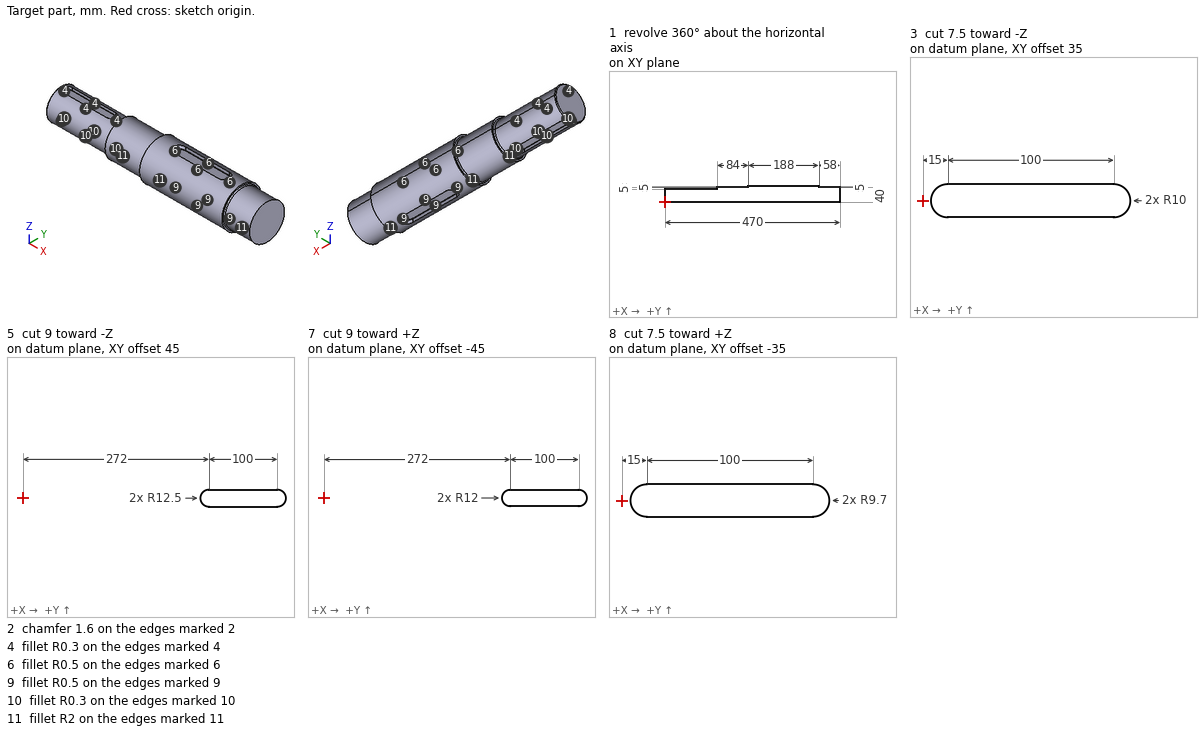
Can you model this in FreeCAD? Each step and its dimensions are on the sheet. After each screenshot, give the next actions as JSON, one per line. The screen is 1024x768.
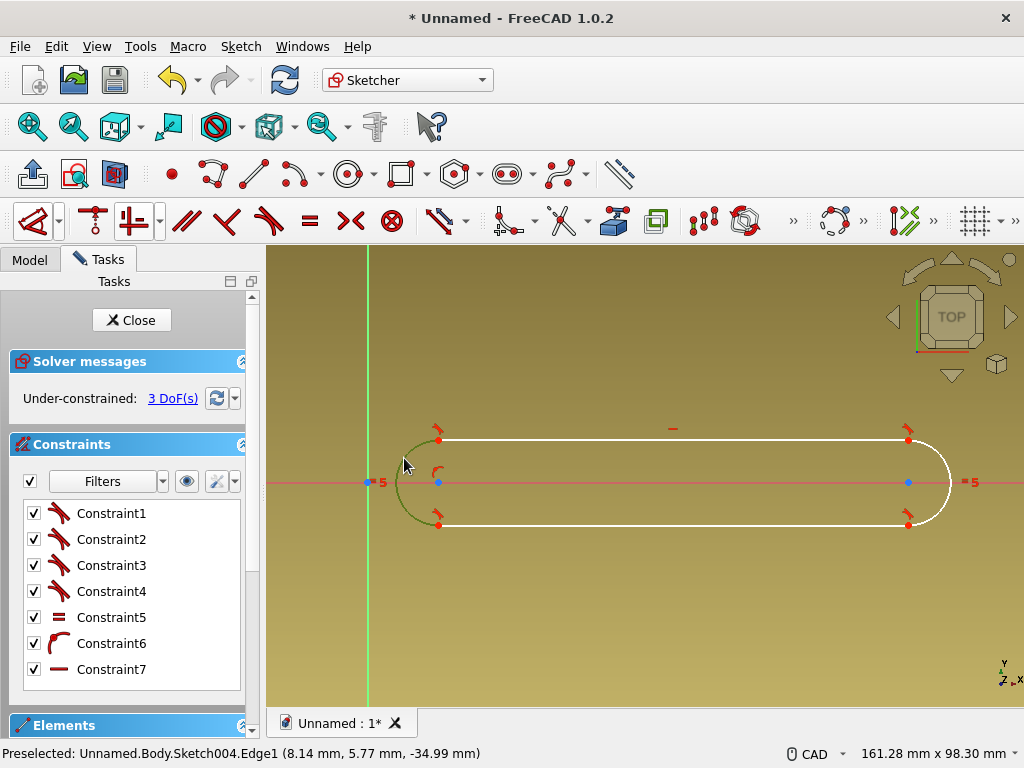
{"action": "left_click", "coordinate": [58, 222]}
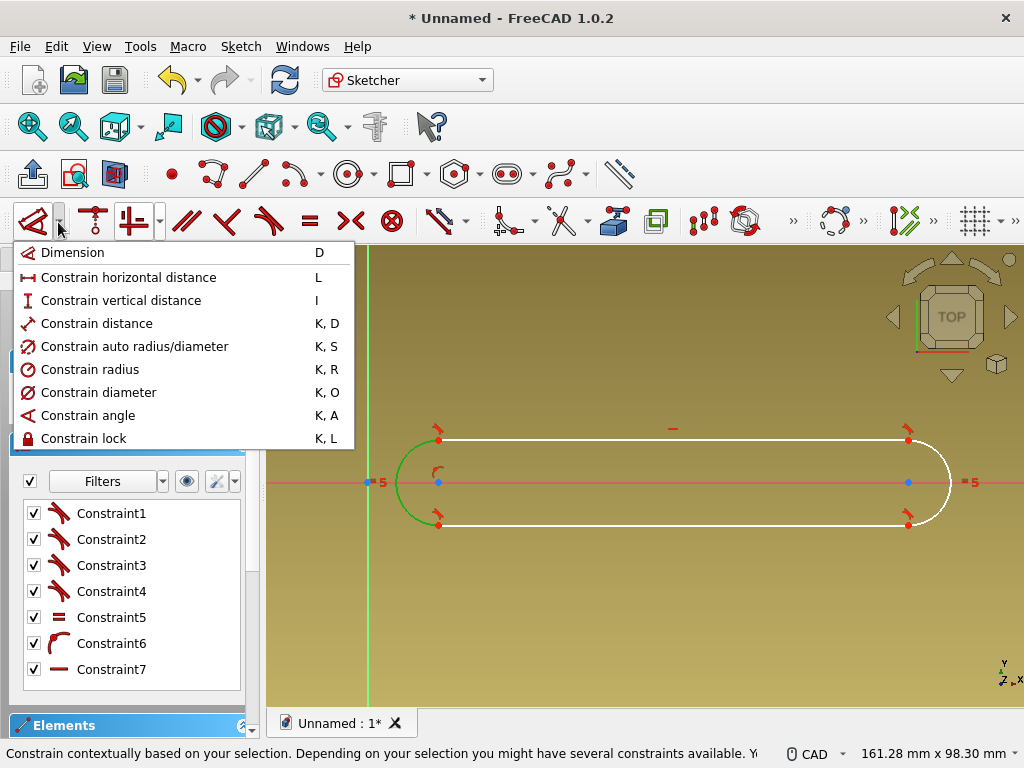
{"action": "left_click", "coordinate": [184, 370]}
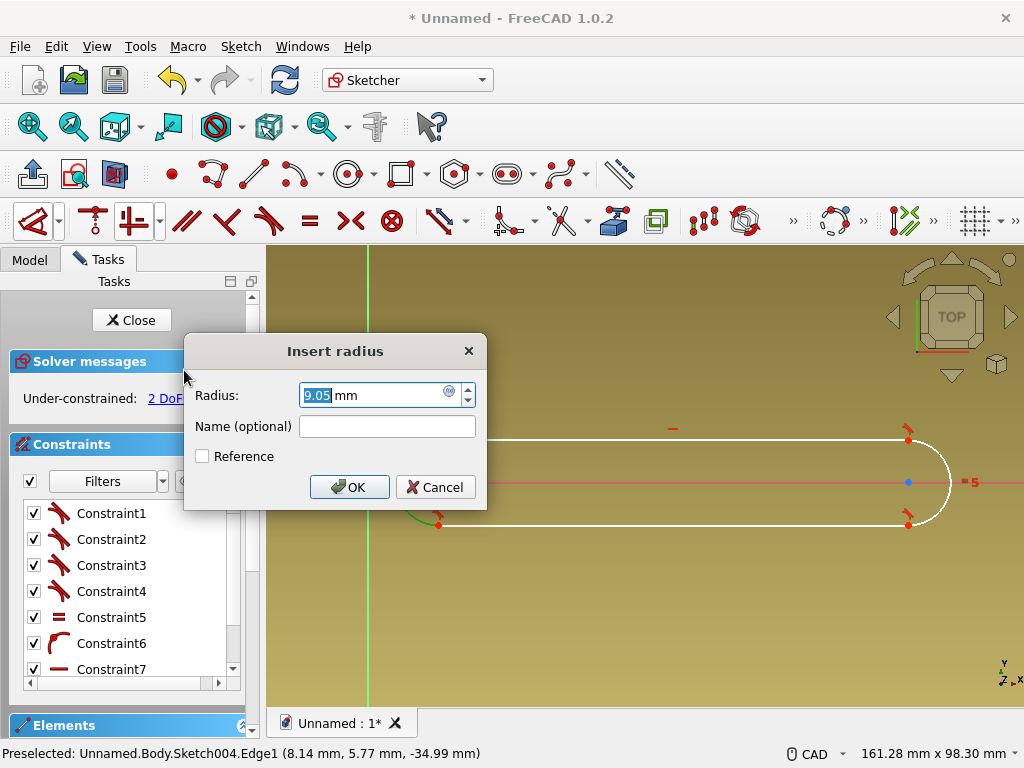
{"action": "type", "text": "9.7"}
{"action": "key", "text": "Return"}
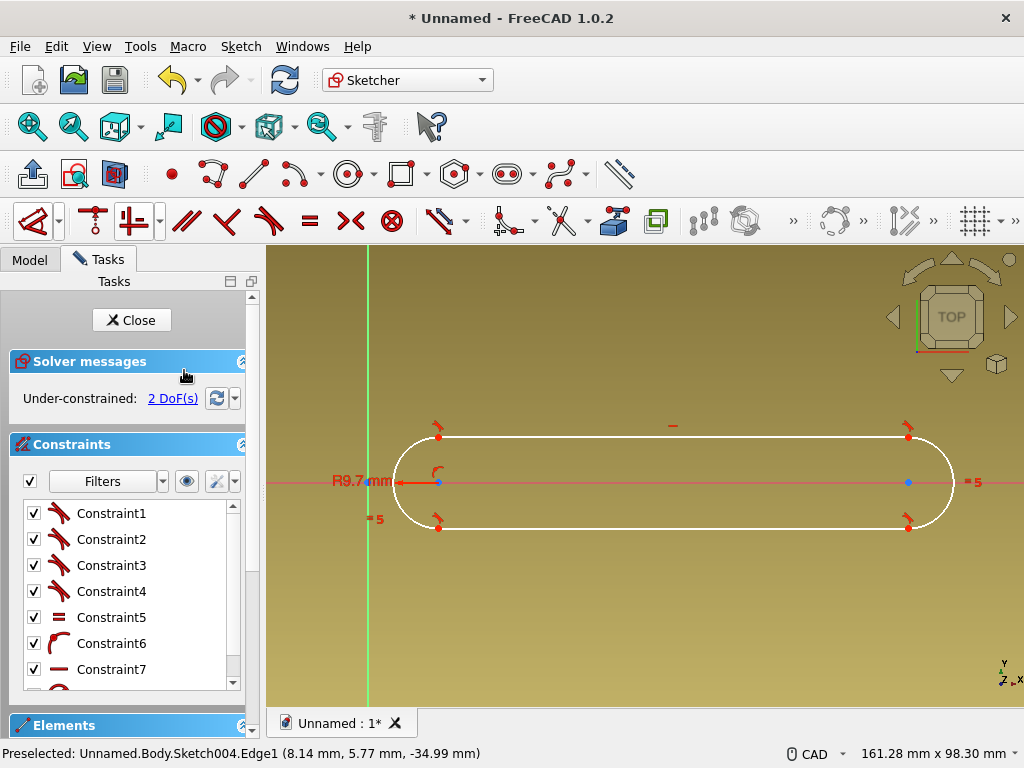
{"action": "left_click", "coordinate": [580, 437]}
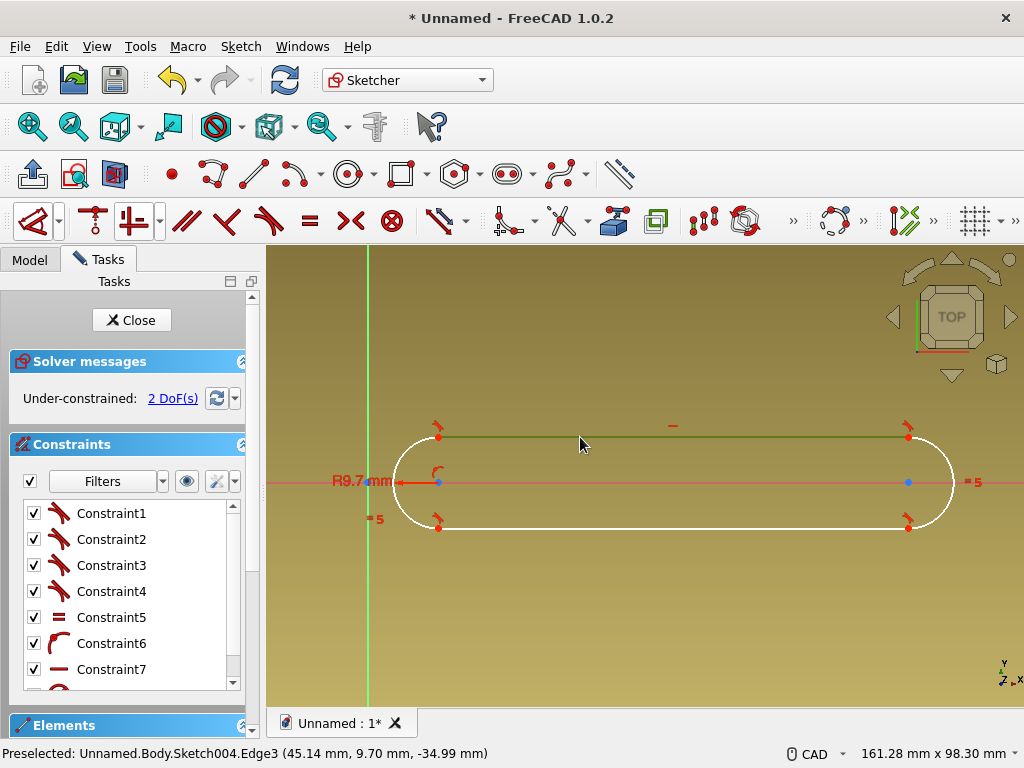
{"action": "left_click", "coordinate": [58, 222]}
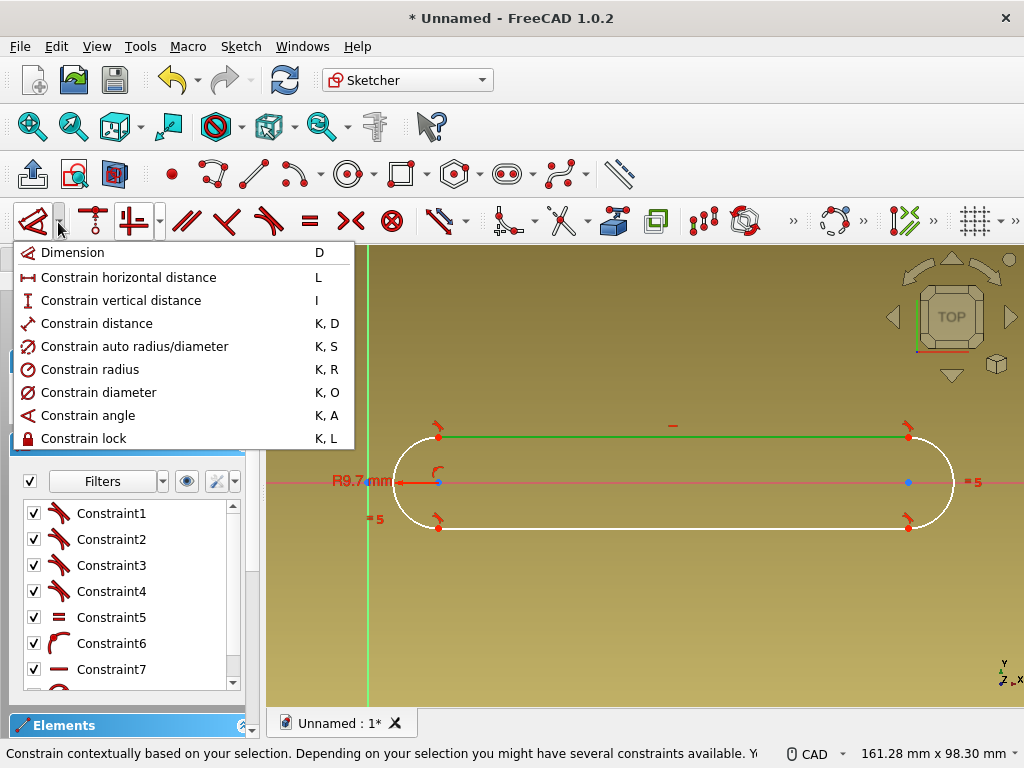
{"action": "left_click", "coordinate": [184, 278]}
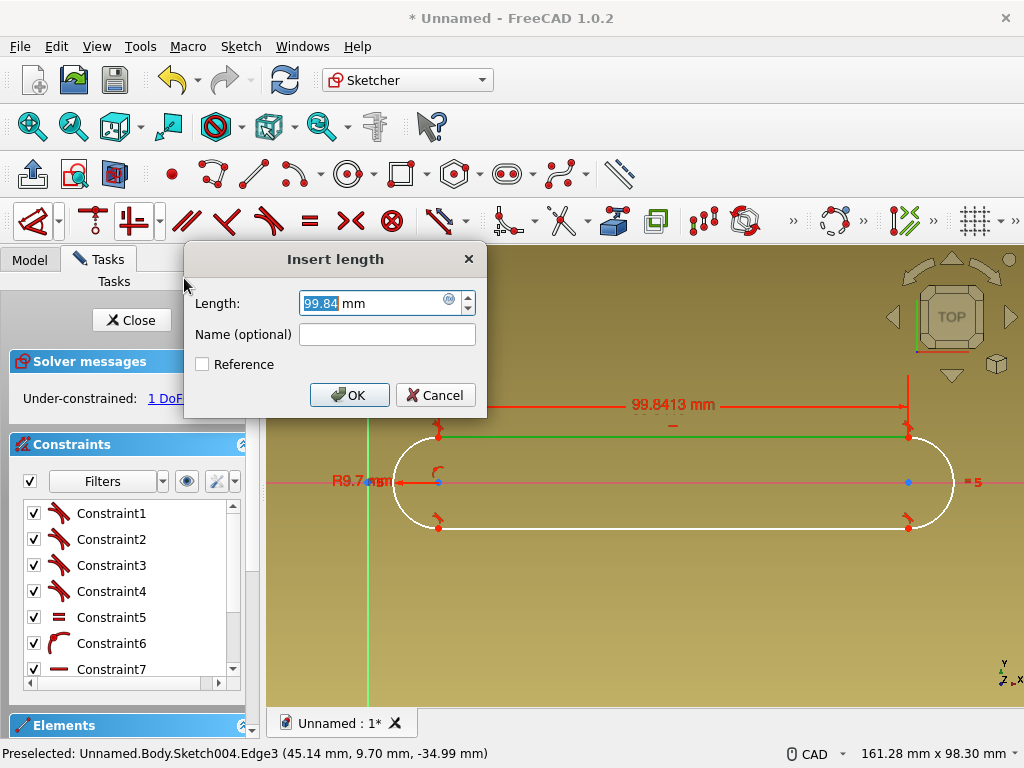
{"action": "type", "text": "100"}
{"action": "key", "text": "Return"}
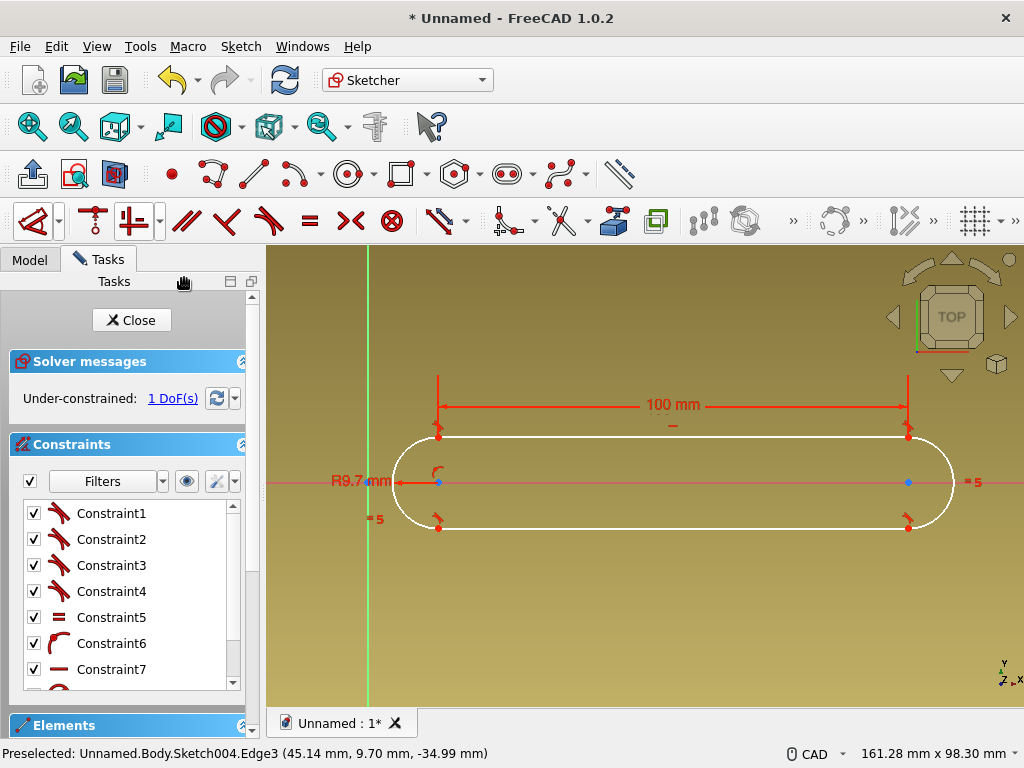
{"action": "left_click", "coordinate": [438, 437]}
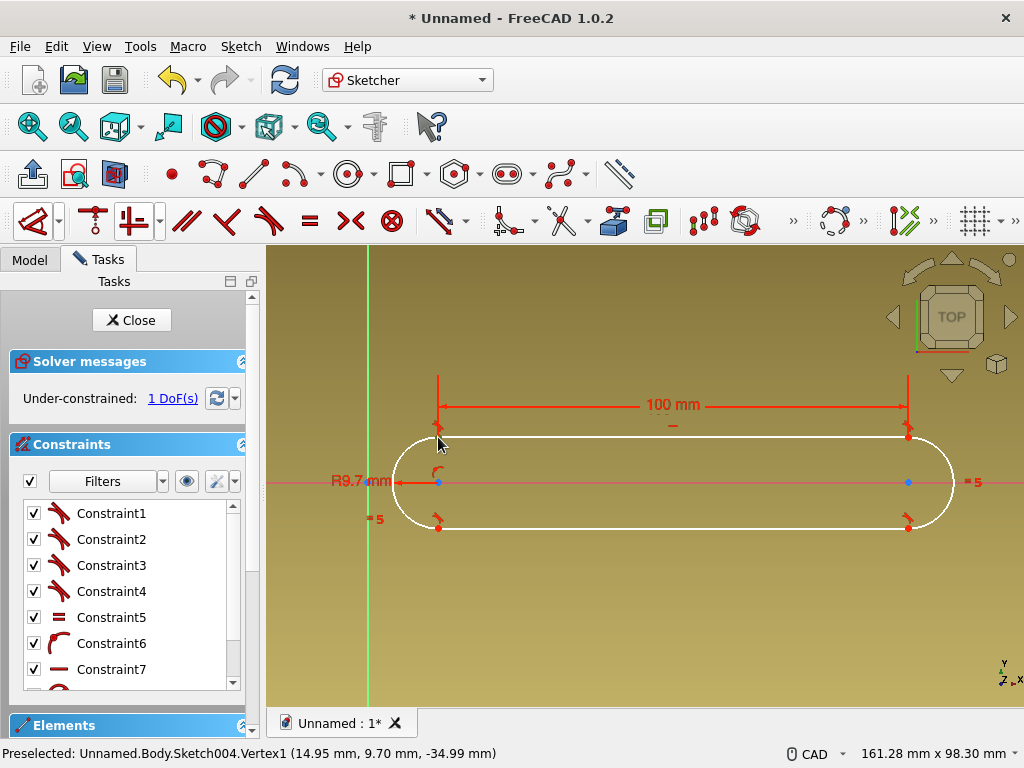
{"action": "key", "text": "l"}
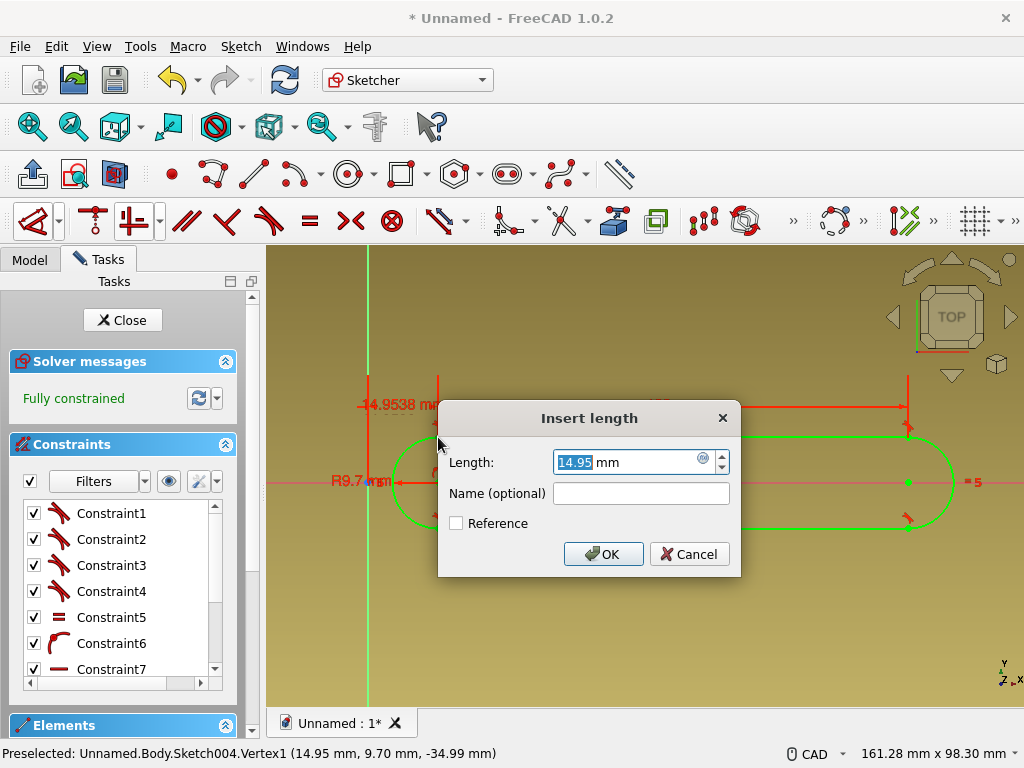
{"action": "type", "text": "15"}
{"action": "key", "text": "Return"}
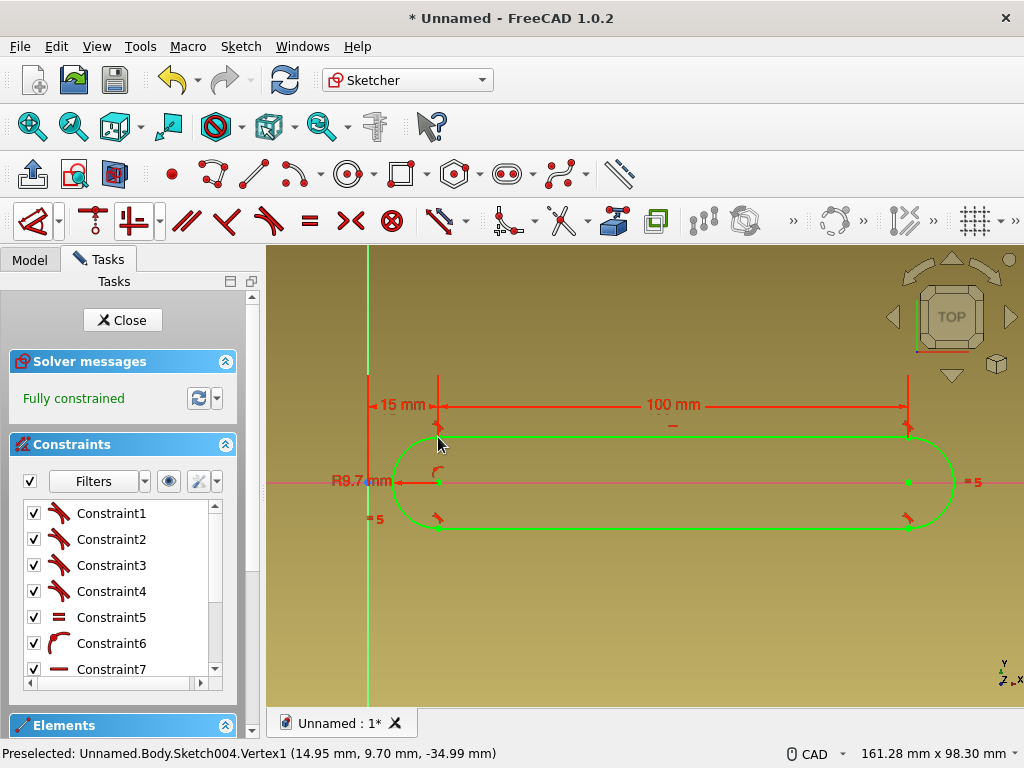
{"action": "left_click", "coordinate": [123, 320]}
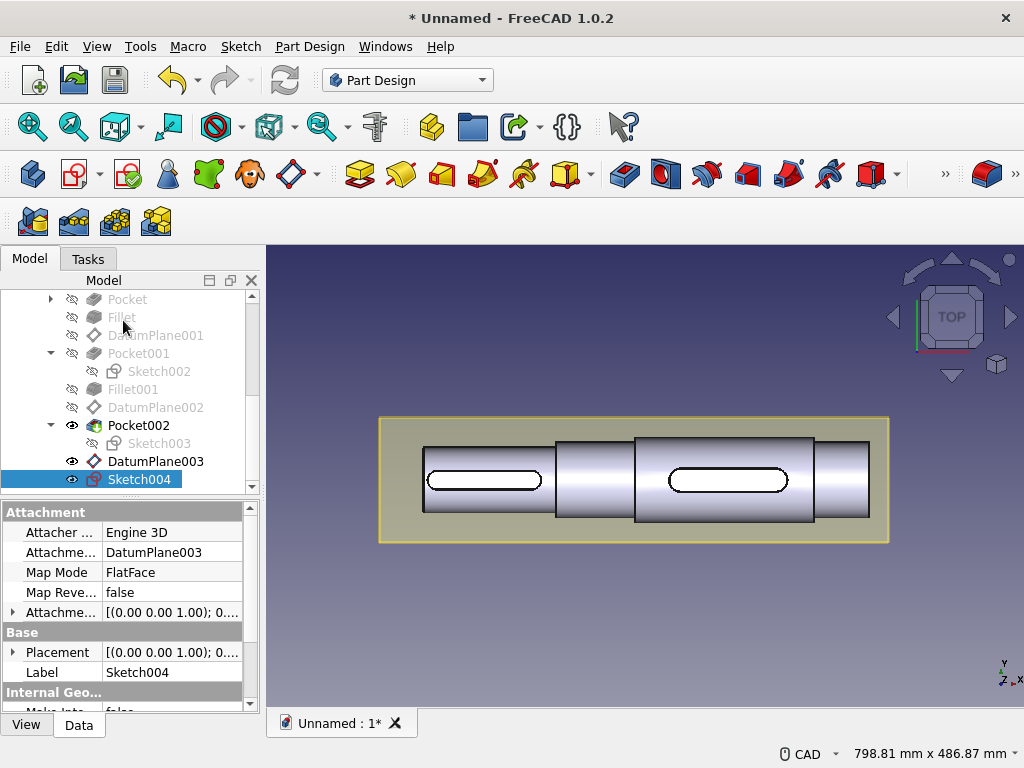
{"action": "left_click", "coordinate": [625, 174]}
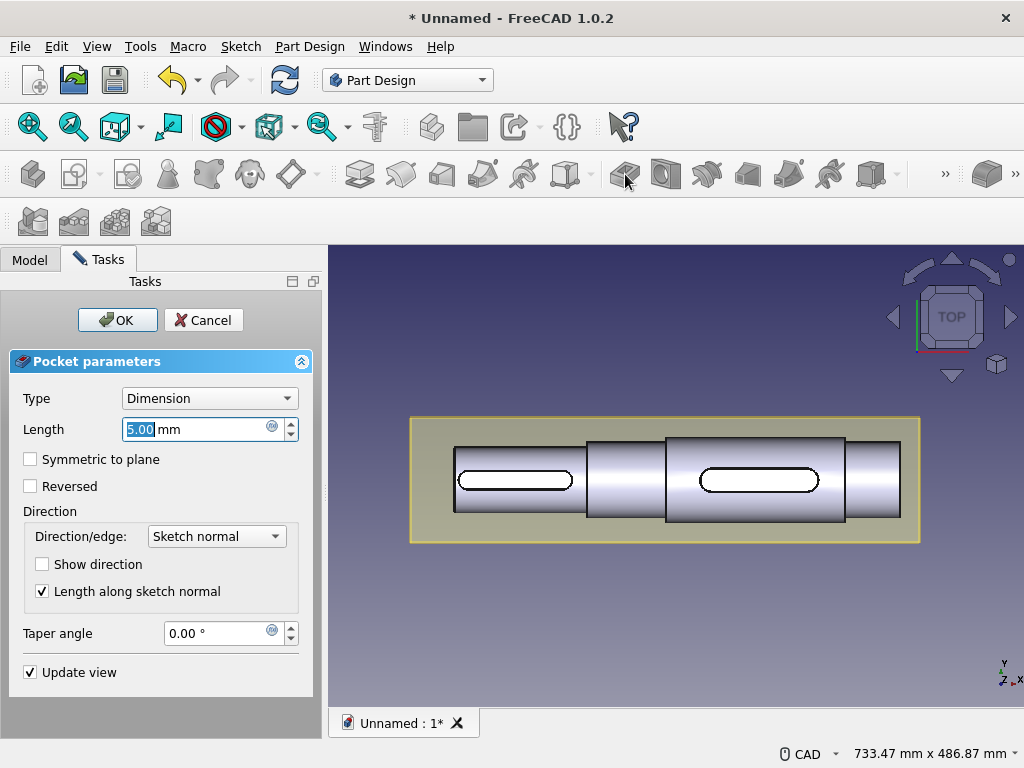
{"action": "type", "text": "7.5"}
{"action": "key", "text": "Tab"}